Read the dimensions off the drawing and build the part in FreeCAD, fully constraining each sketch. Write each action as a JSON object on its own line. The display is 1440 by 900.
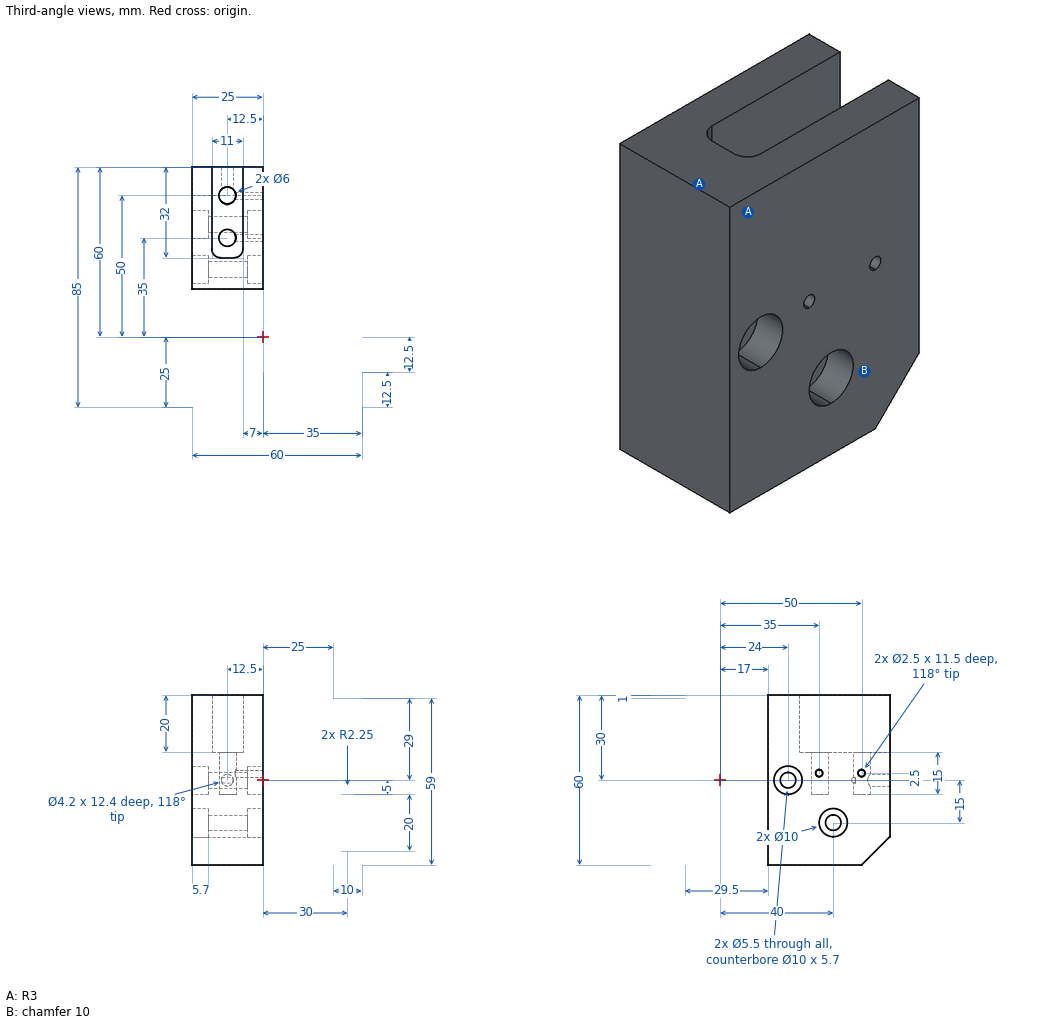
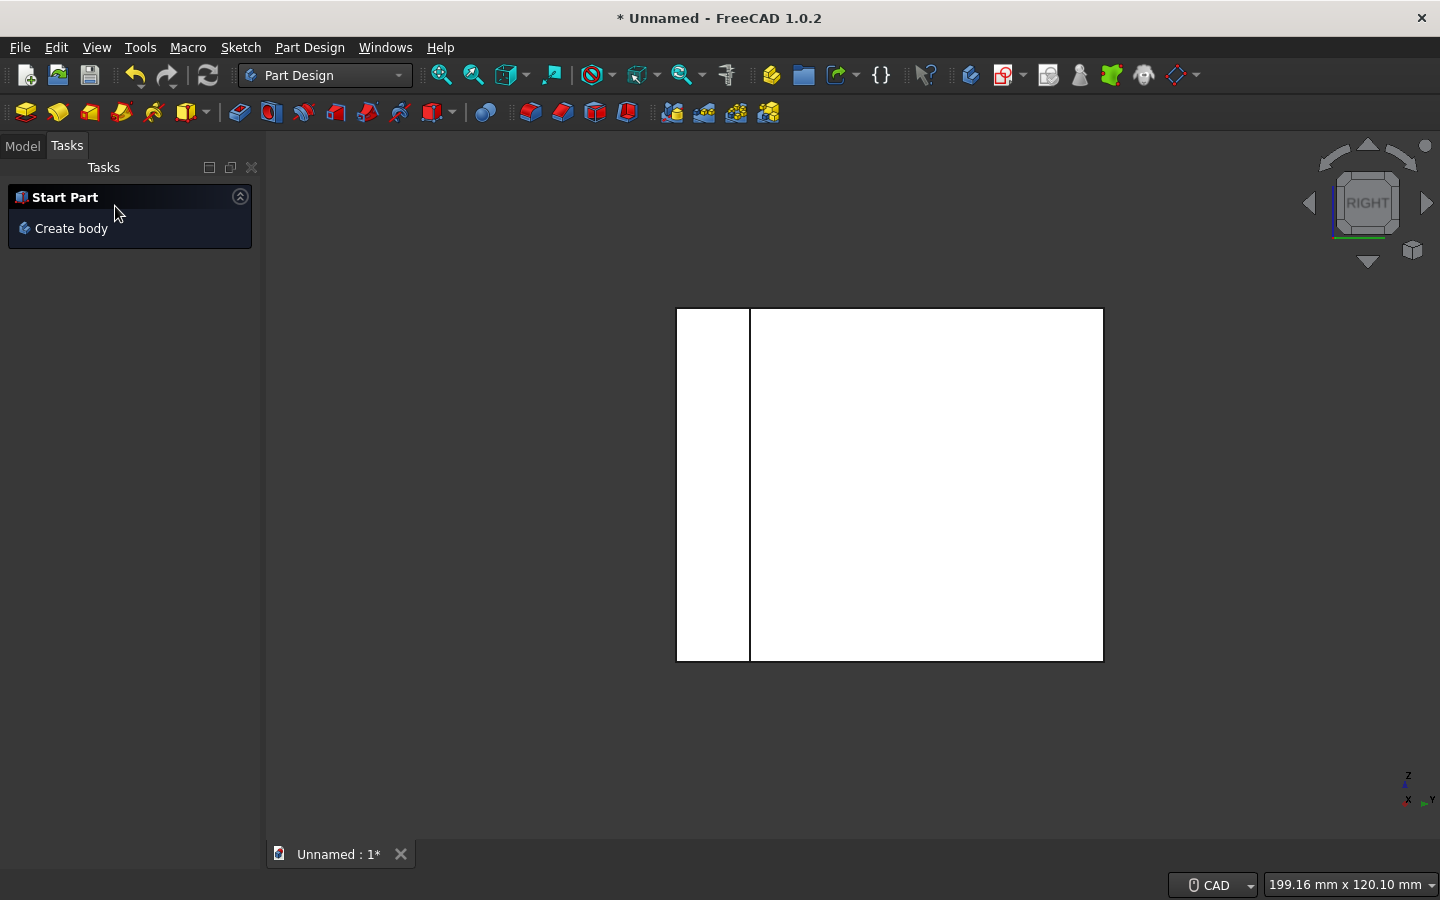
{"action": "key", "text": "5"}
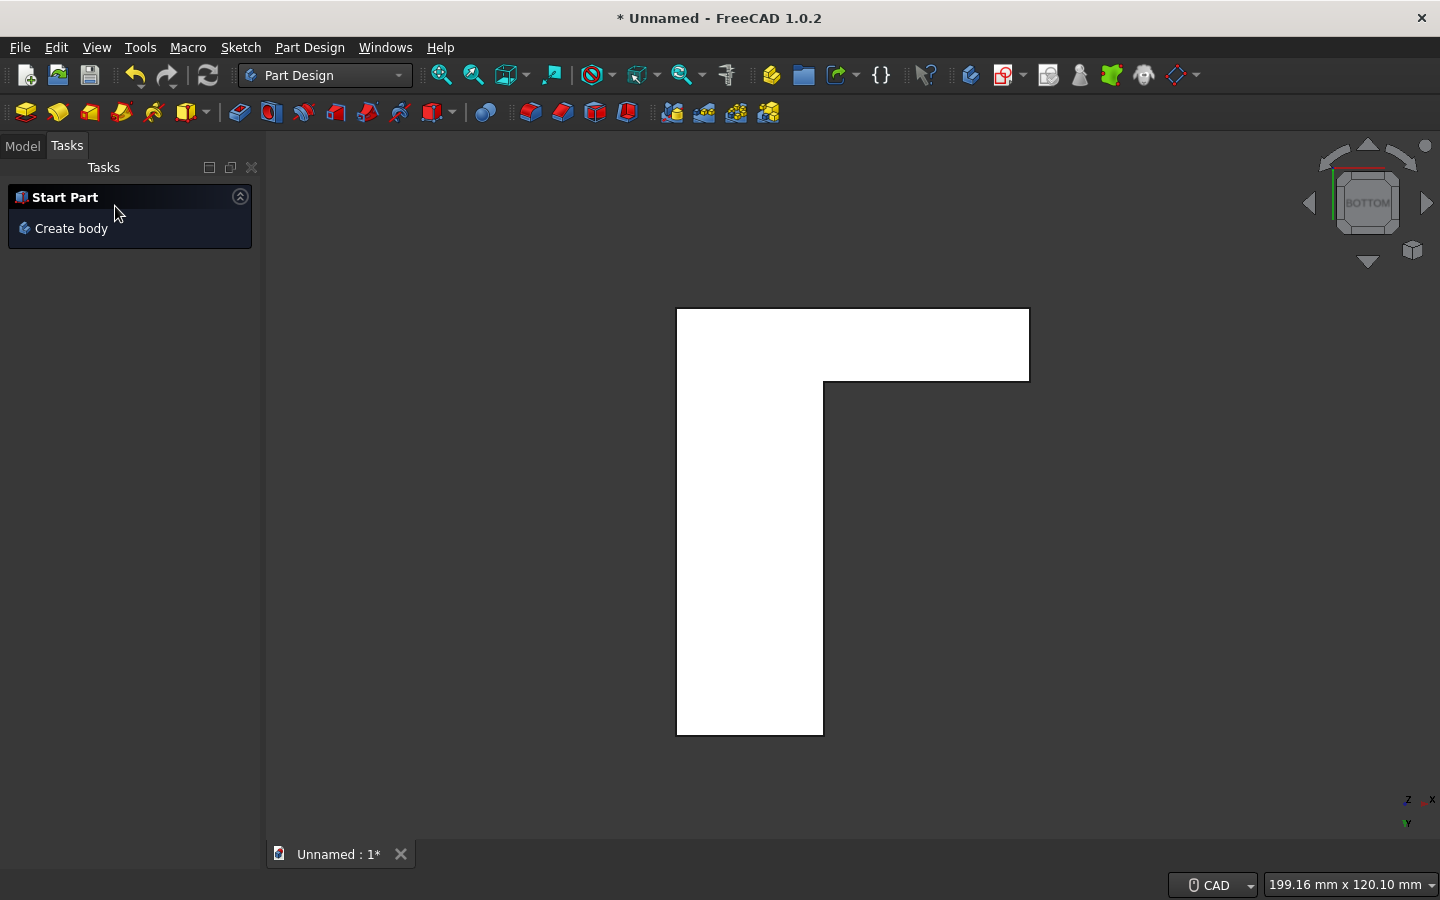
{"action": "key", "text": "4"}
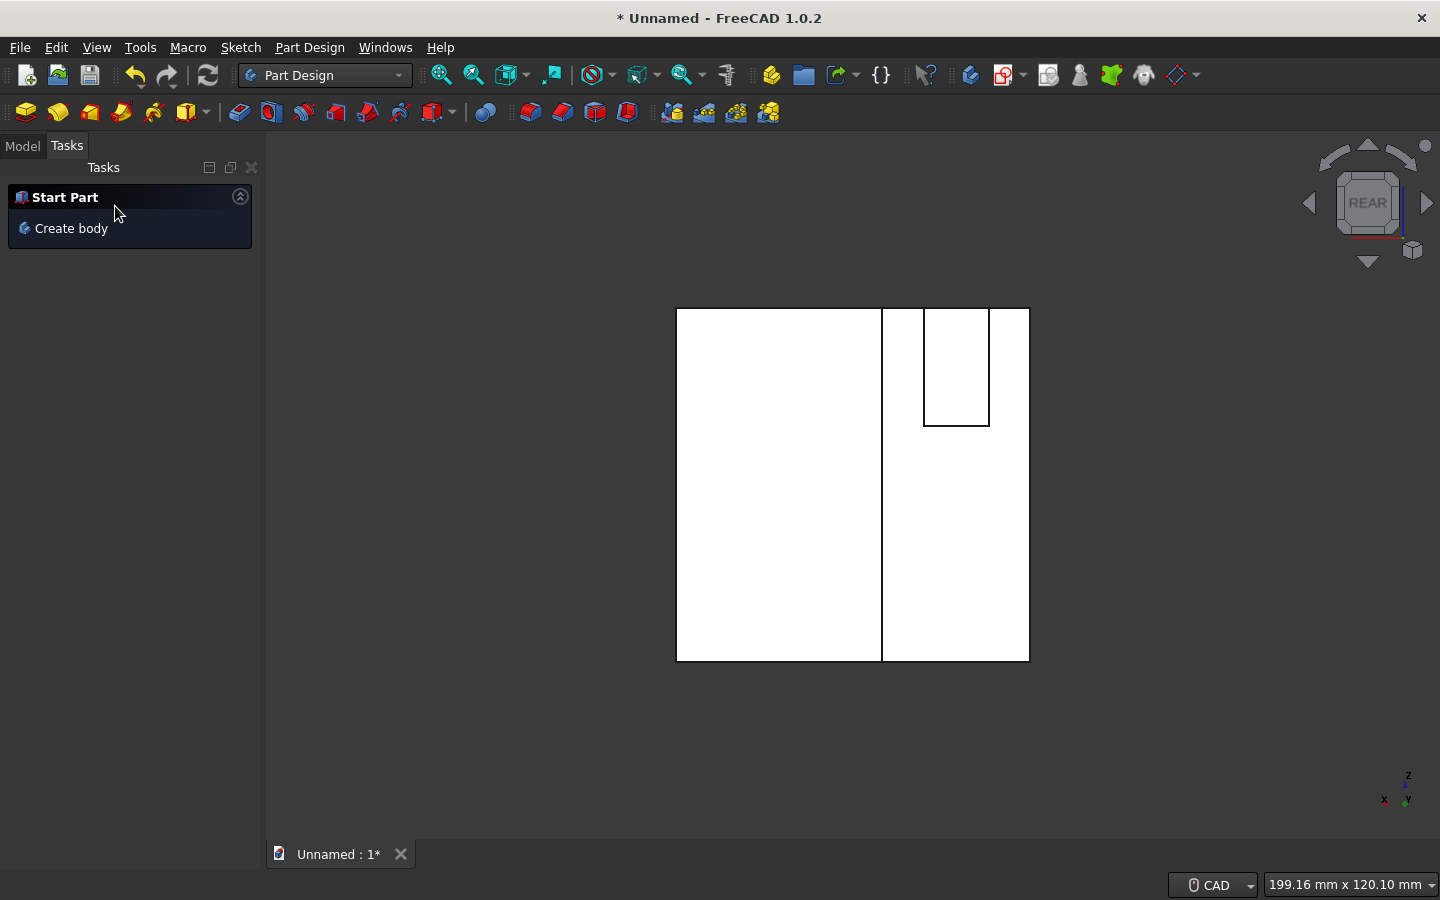
{"action": "key", "text": "6"}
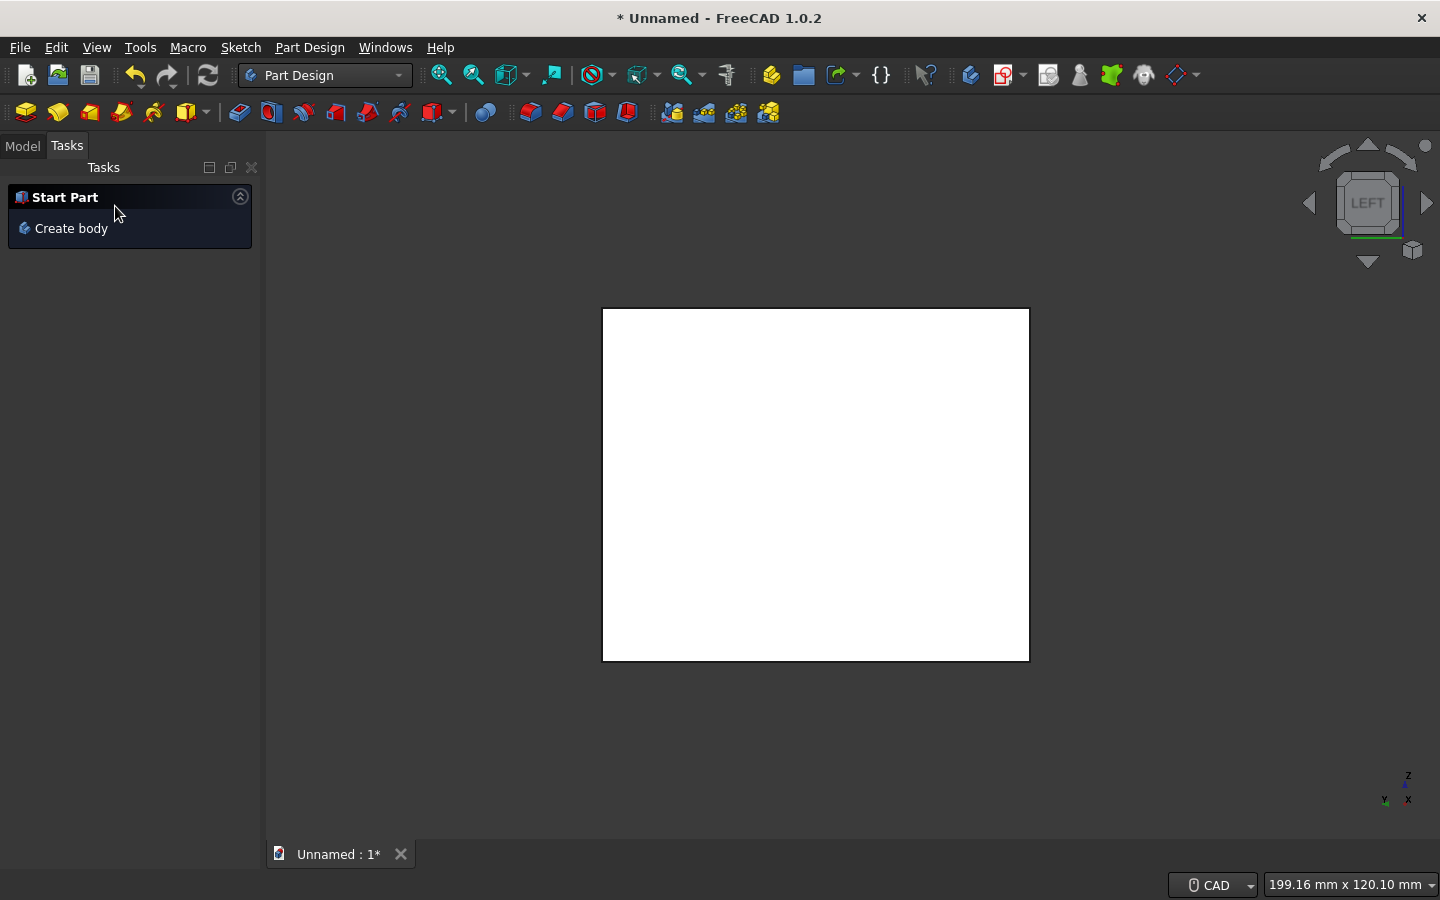
{"action": "key", "text": "v 3"}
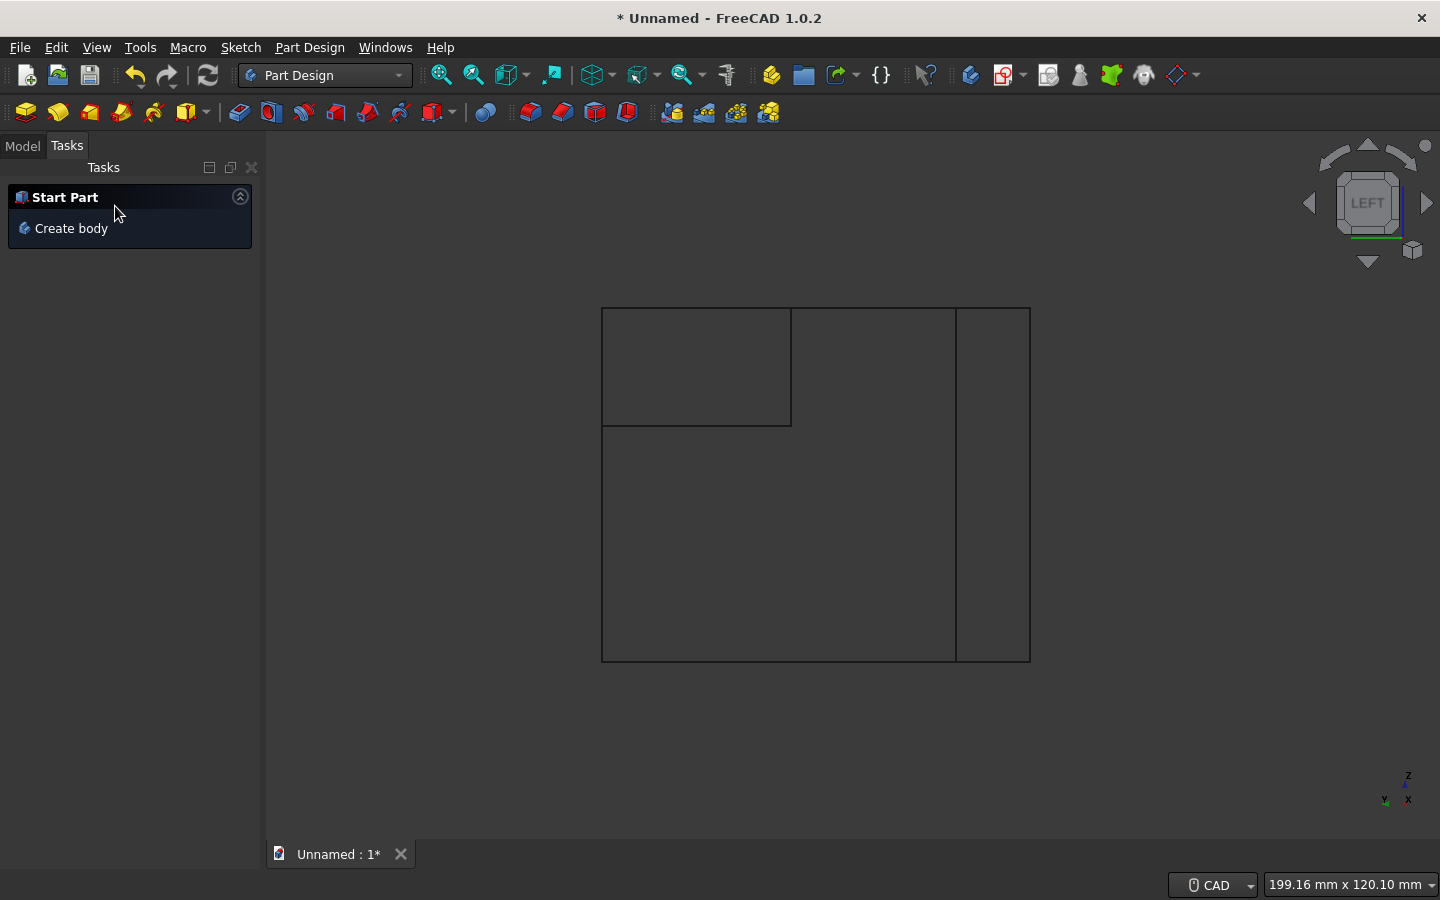
{"action": "key", "text": "0"}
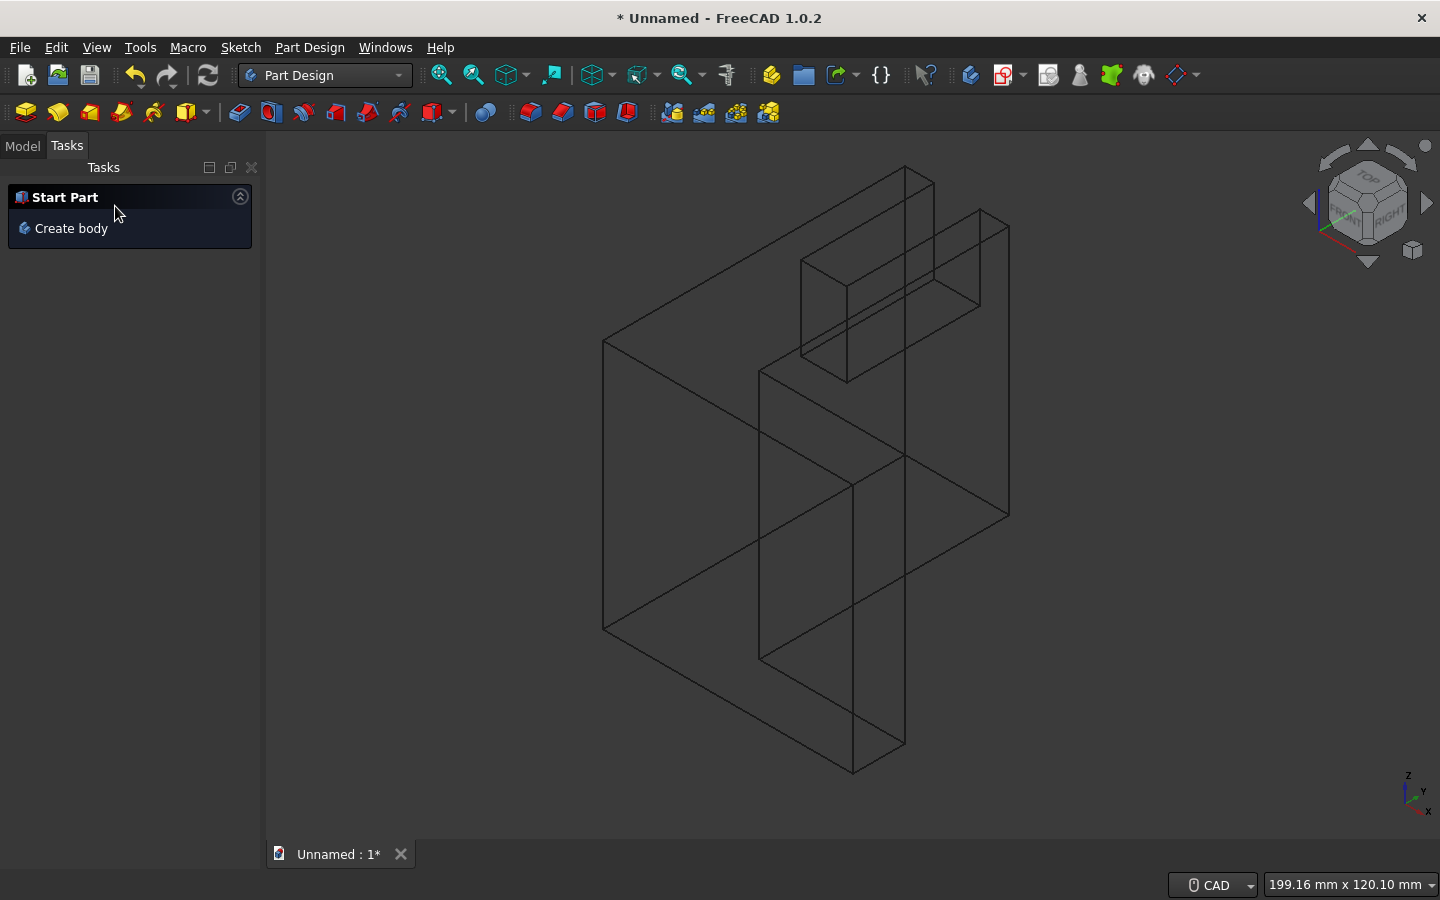
{"action": "left_click", "coordinate": [847, 334]}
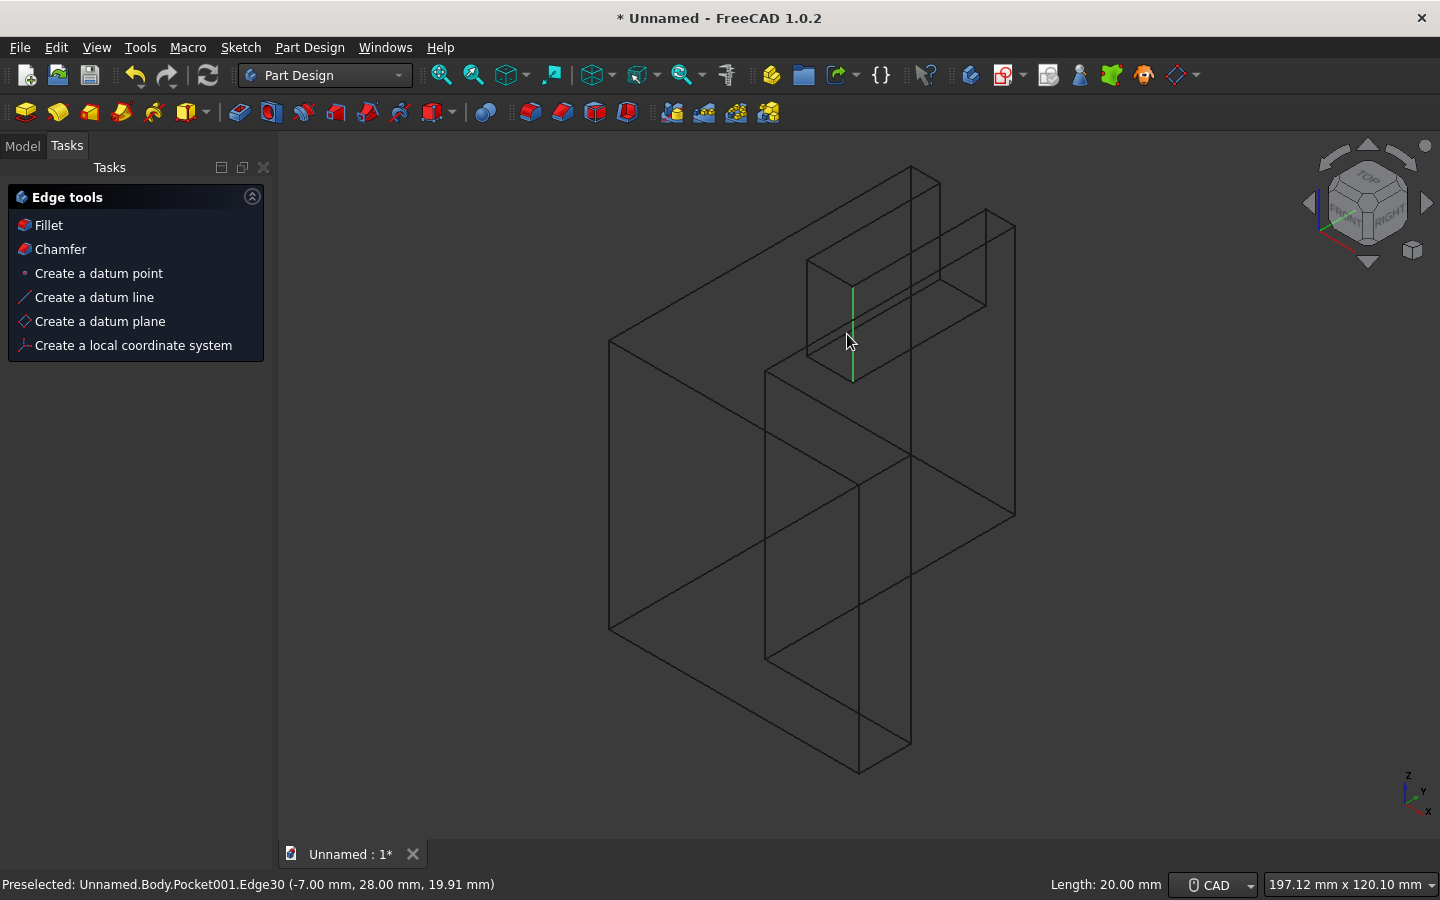
{"action": "left_click", "coordinate": [807, 307], "text": "ctrl"}